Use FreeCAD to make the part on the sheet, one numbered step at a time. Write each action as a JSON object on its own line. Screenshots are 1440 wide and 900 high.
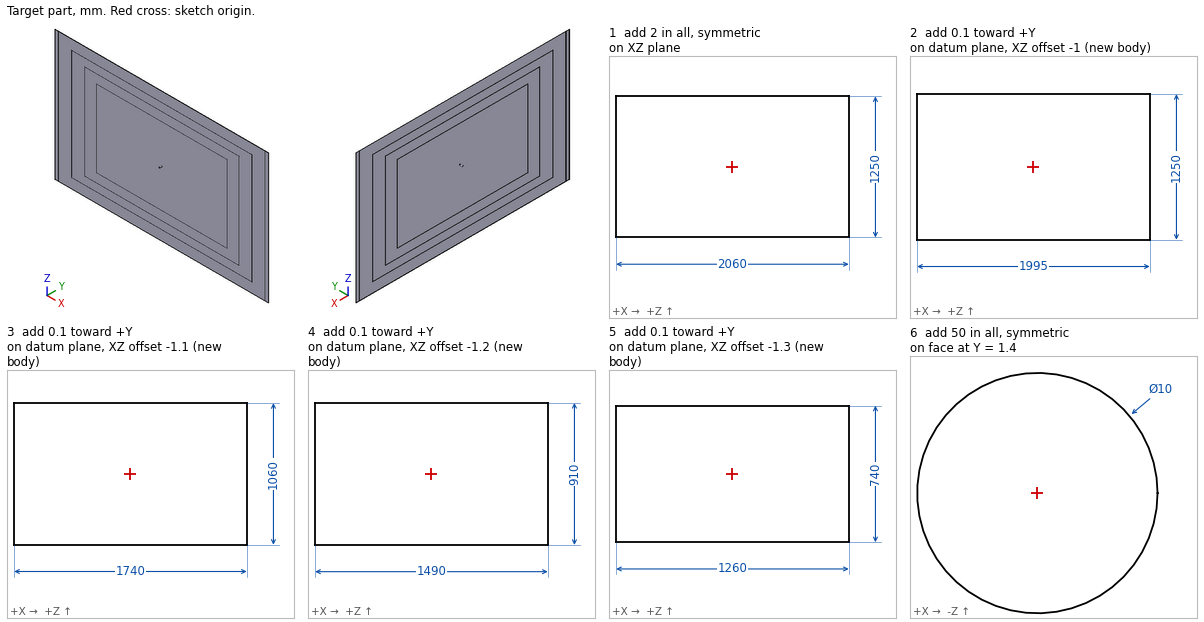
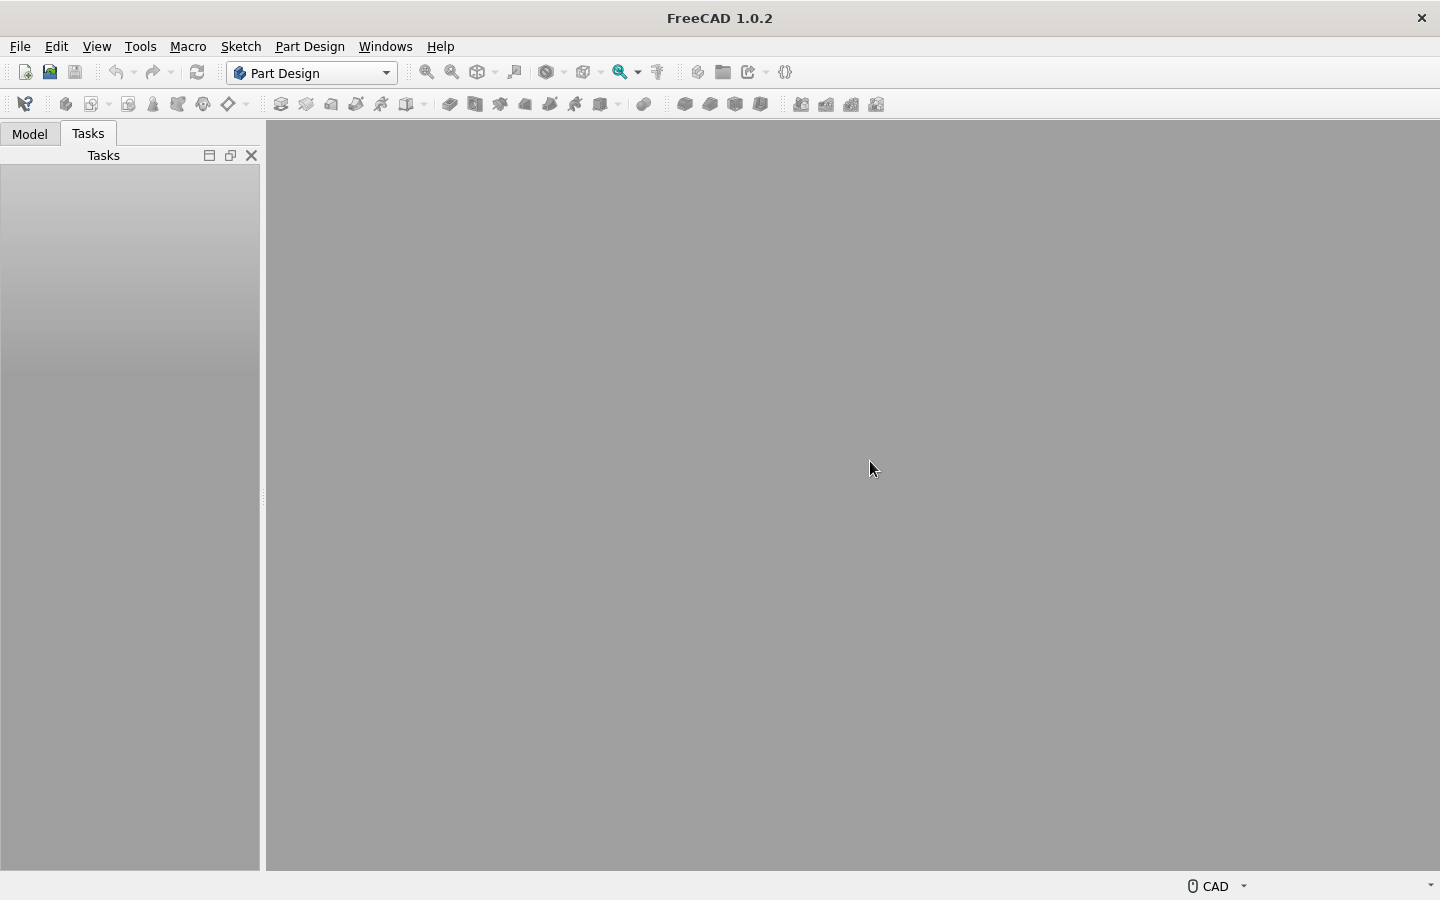
{"action": "left_click", "coordinate": [25, 72]}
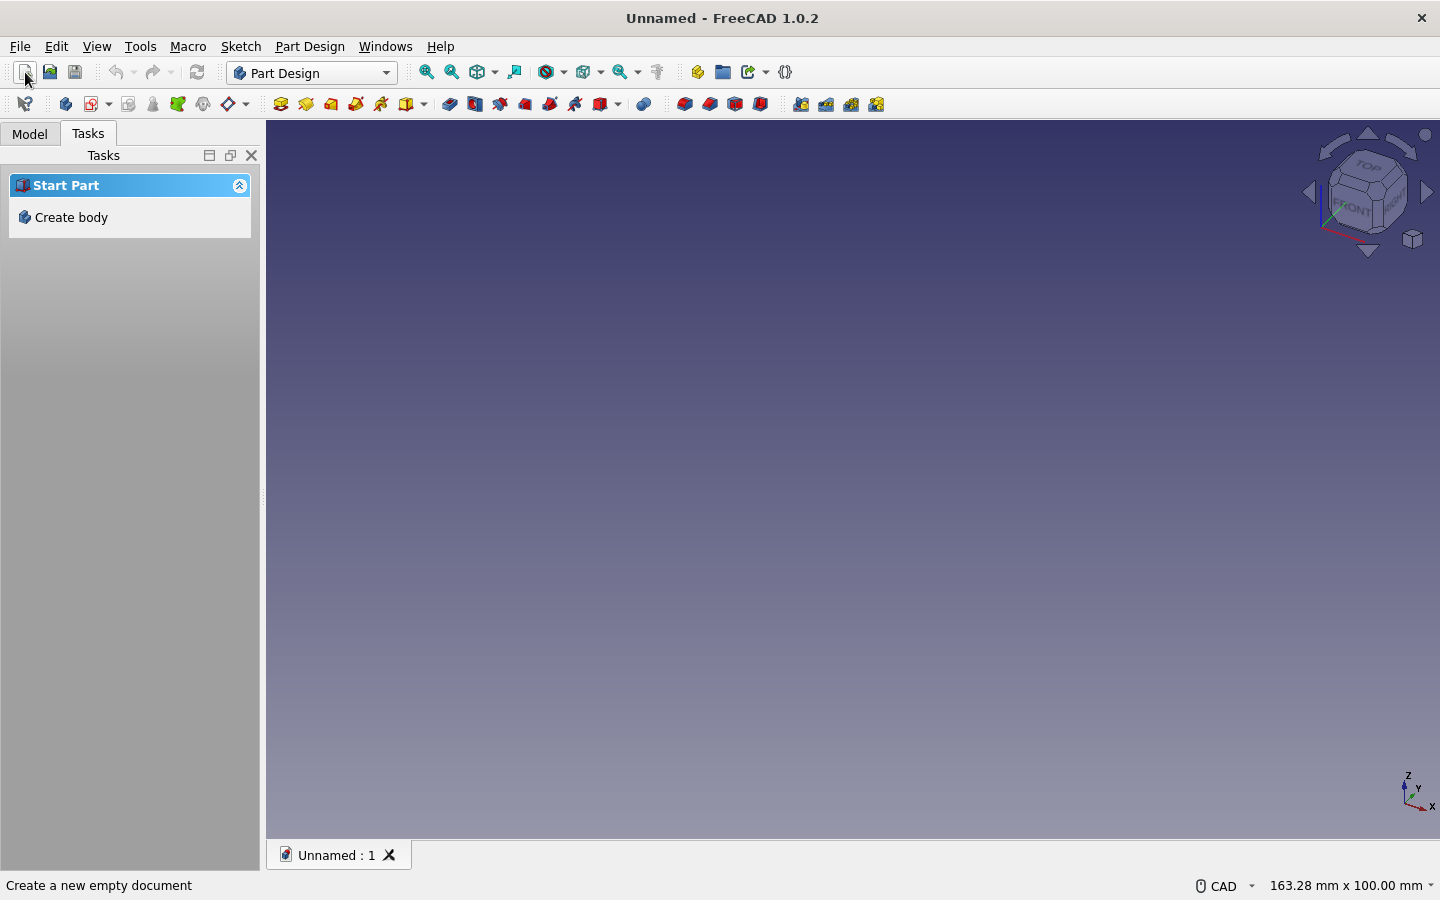
{"action": "left_click", "coordinate": [90, 104]}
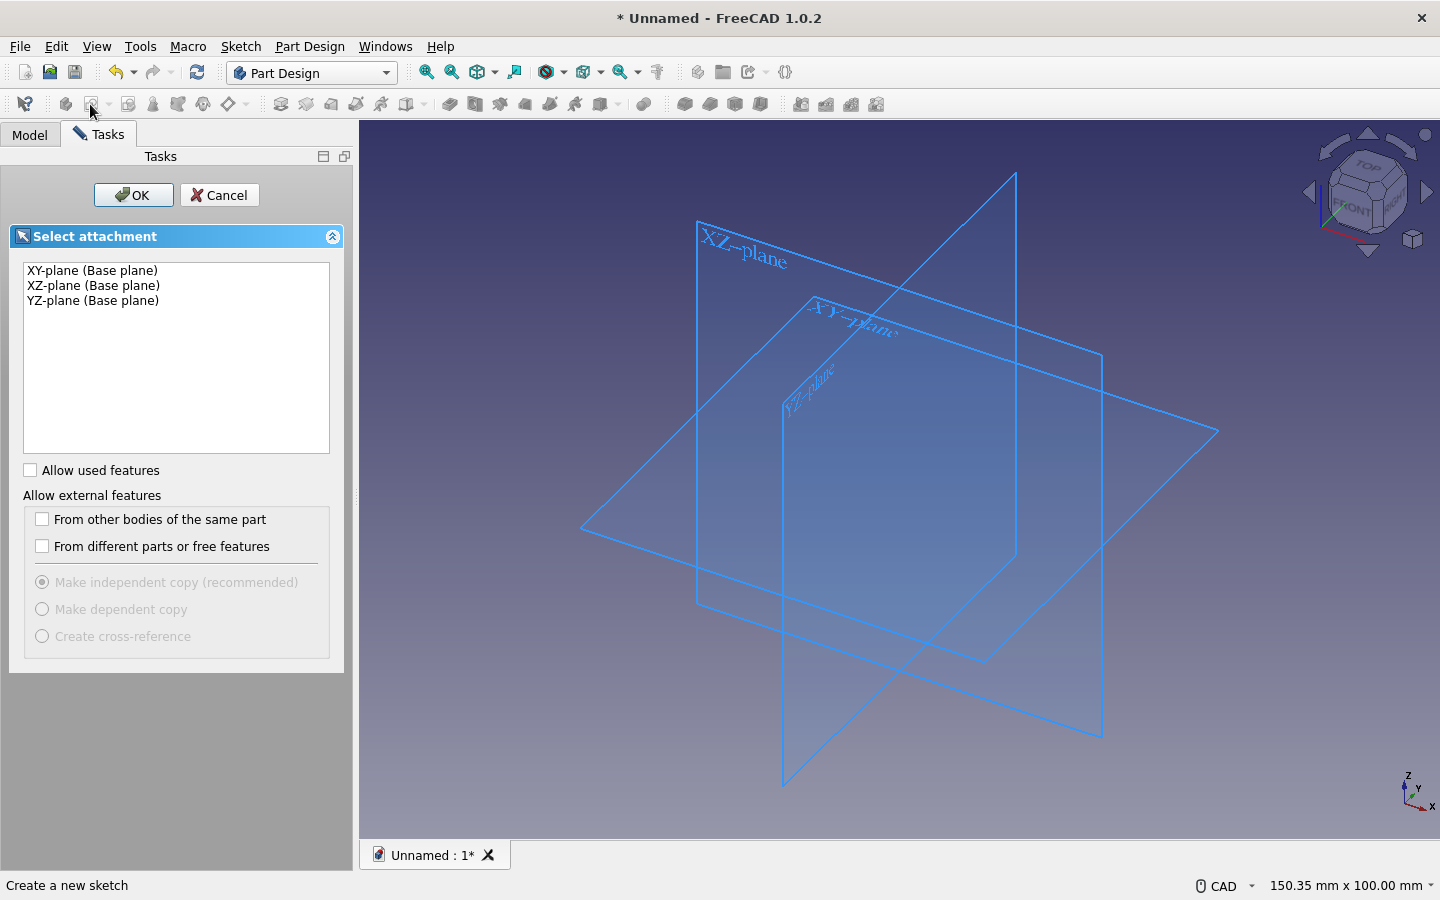
{"action": "left_click", "coordinate": [84, 286]}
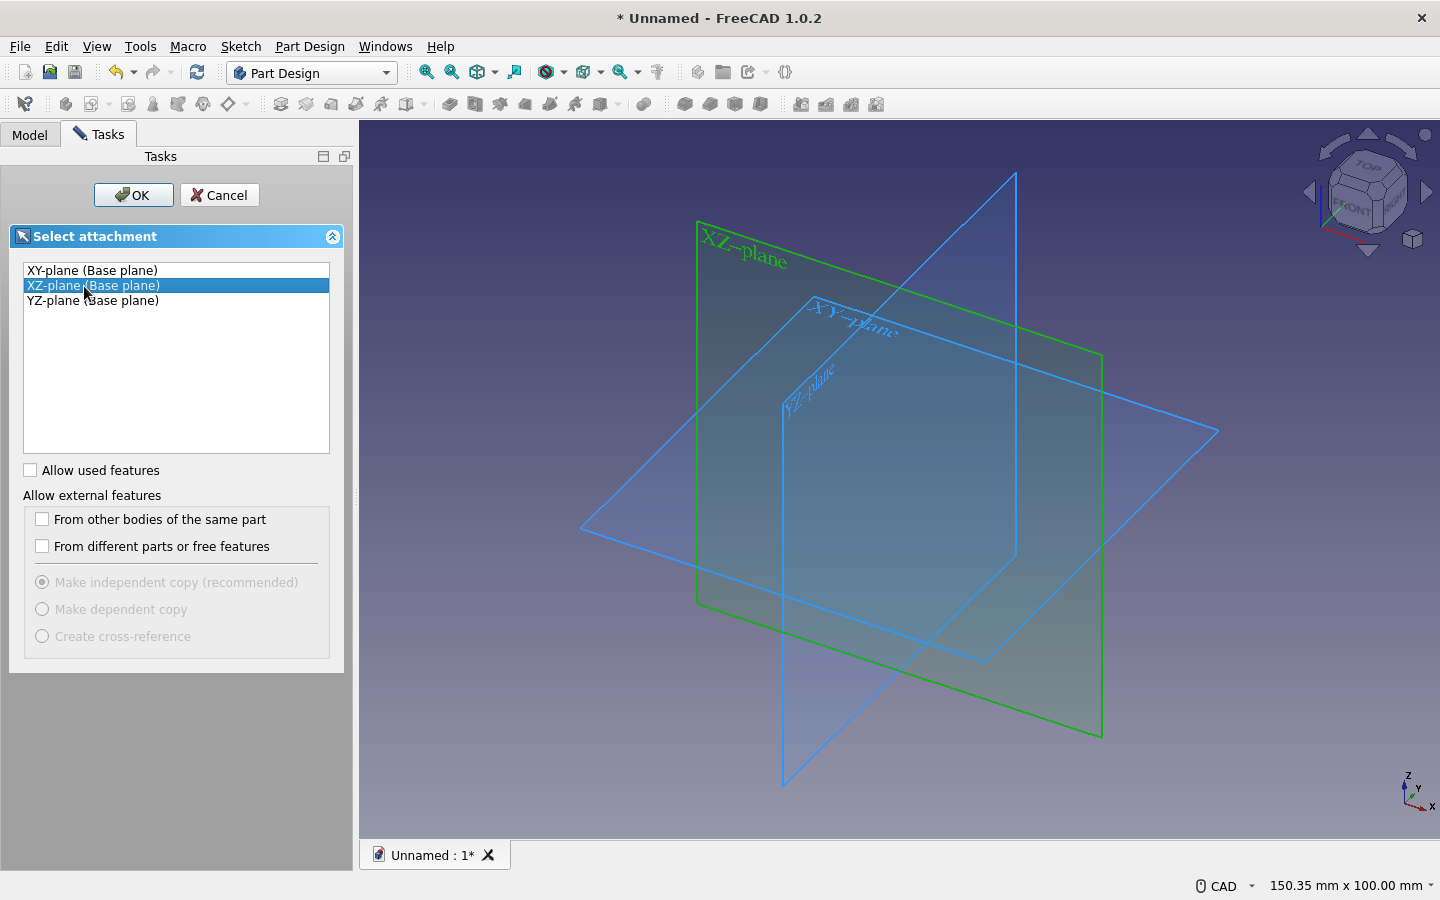
{"action": "left_click", "coordinate": [134, 195]}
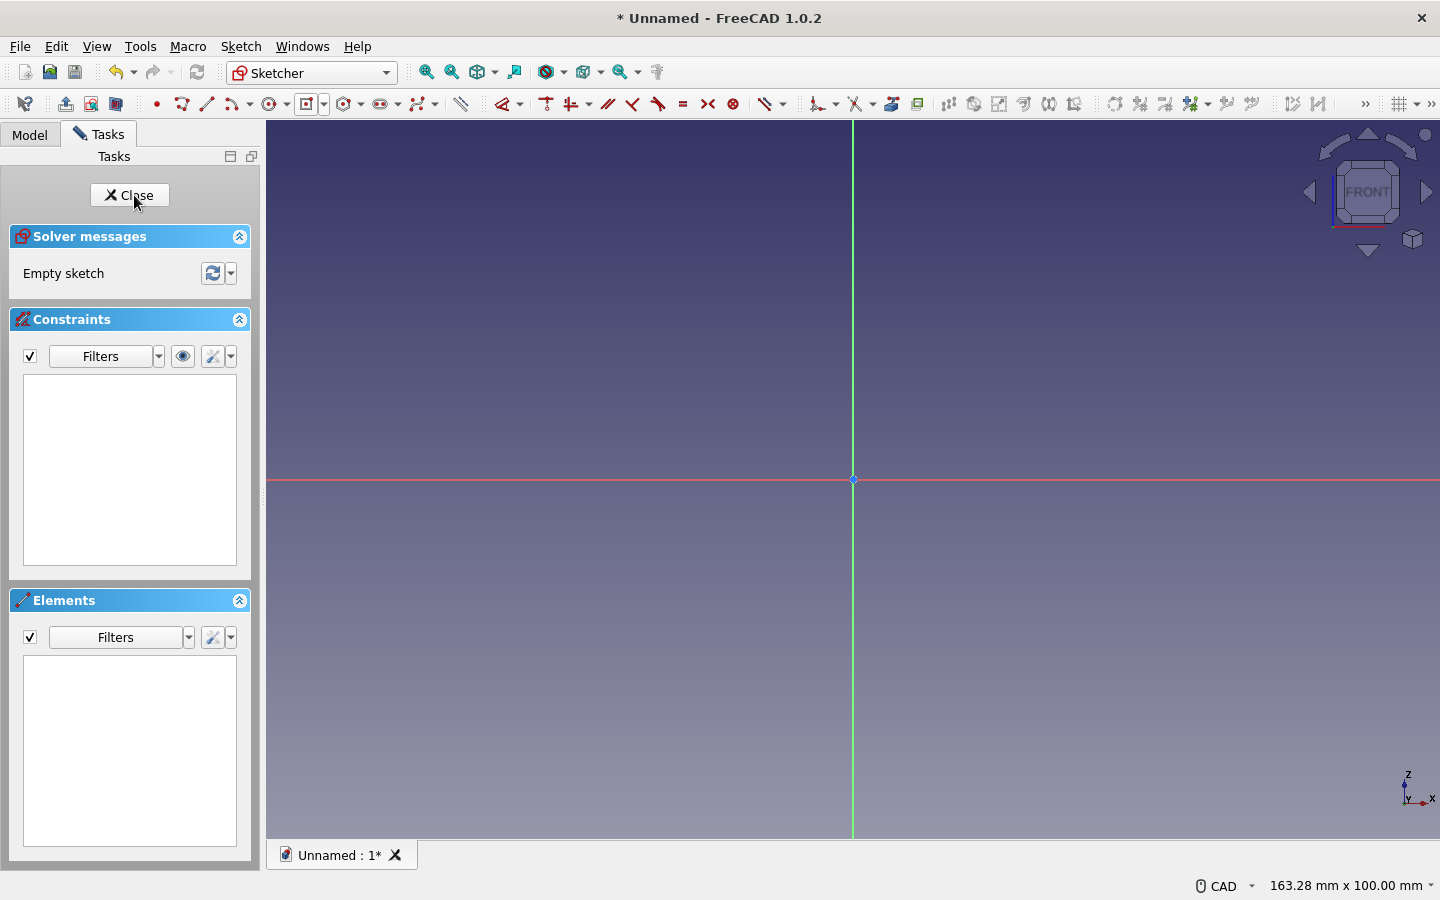
{"action": "scroll", "coordinate": [781, 480], "scroll_direction": "down", "scroll_amount": 15}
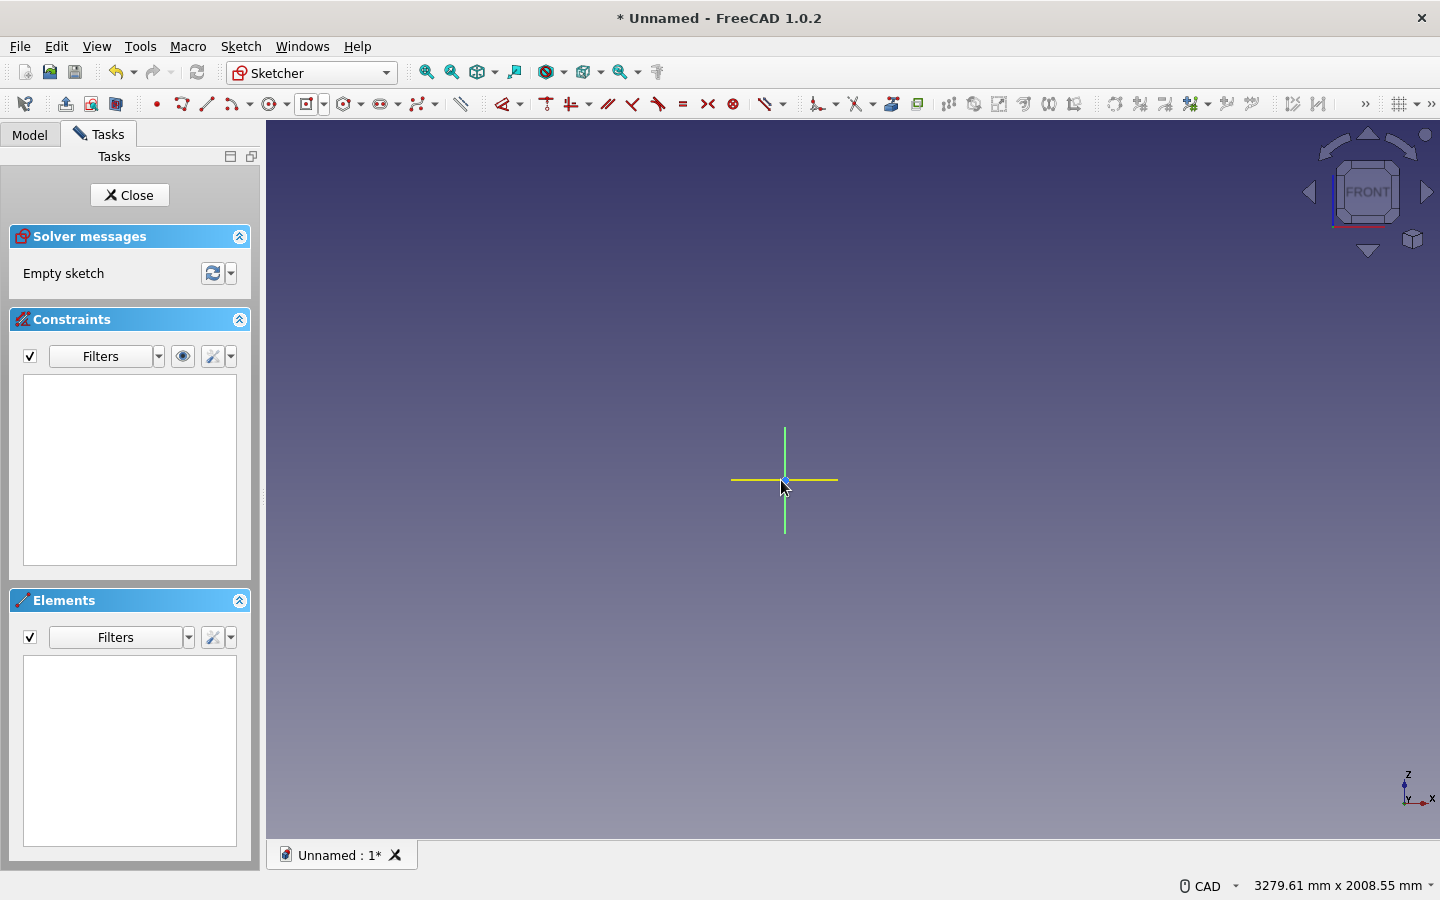
{"action": "left_click", "coordinate": [306, 104]}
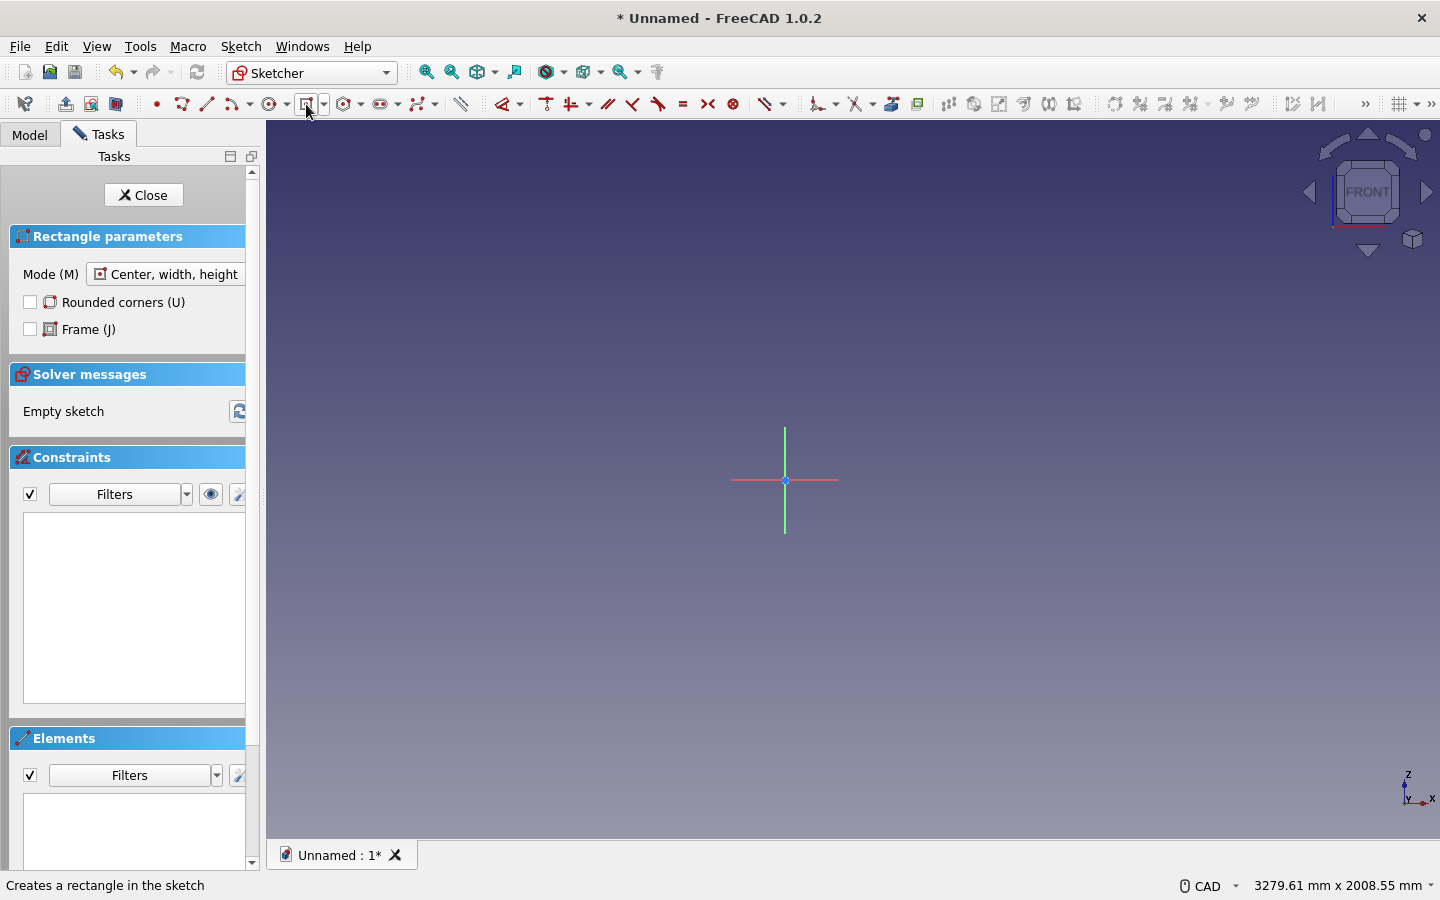
{"action": "left_click", "coordinate": [785, 480]}
{"action": "mouse_move", "coordinate": [1154, 257]}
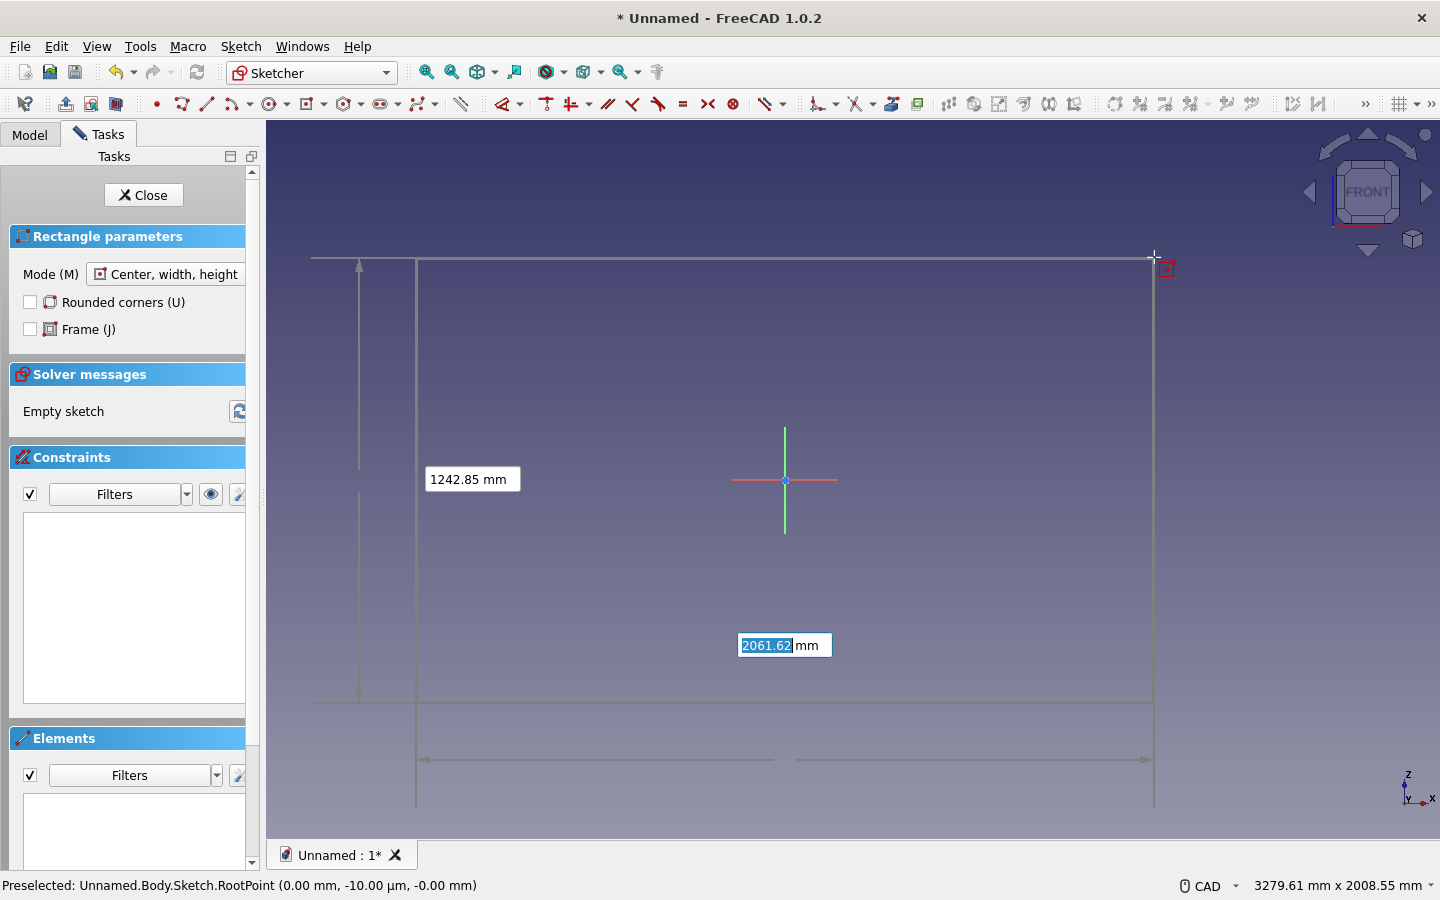
{"action": "type", "text": "2060"}
{"action": "key", "text": "Tab"}
{"action": "type", "text": "1250"}
{"action": "key", "text": "Return"}
{"action": "key", "text": "Escape"}